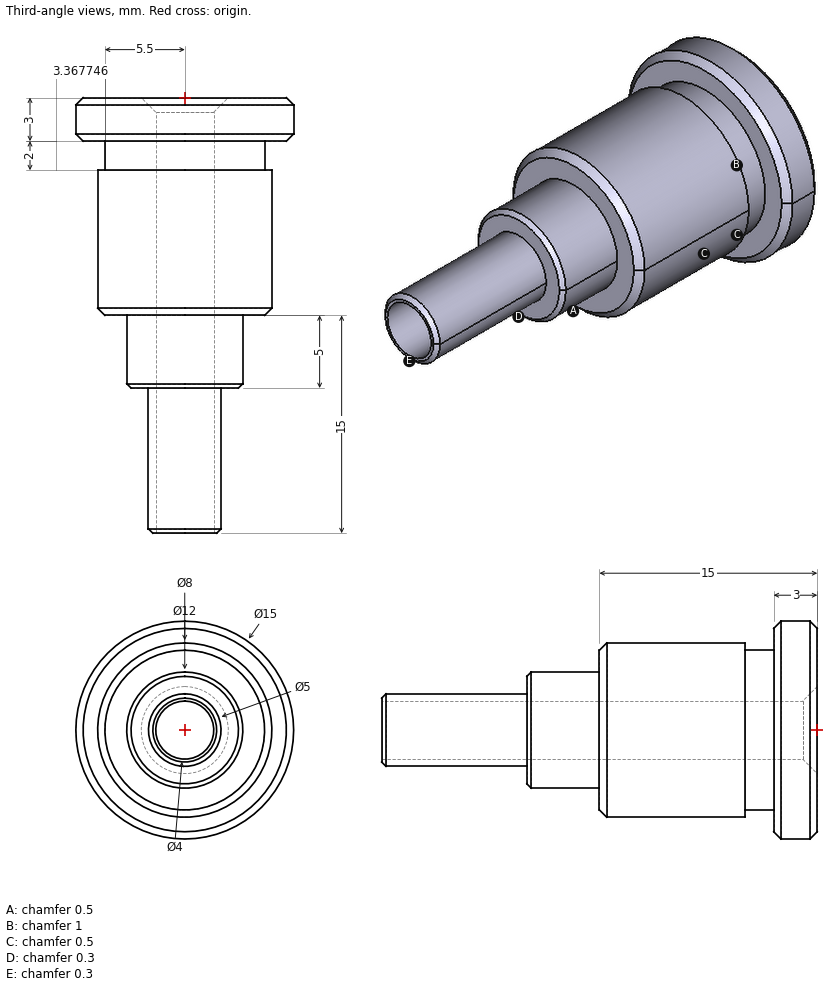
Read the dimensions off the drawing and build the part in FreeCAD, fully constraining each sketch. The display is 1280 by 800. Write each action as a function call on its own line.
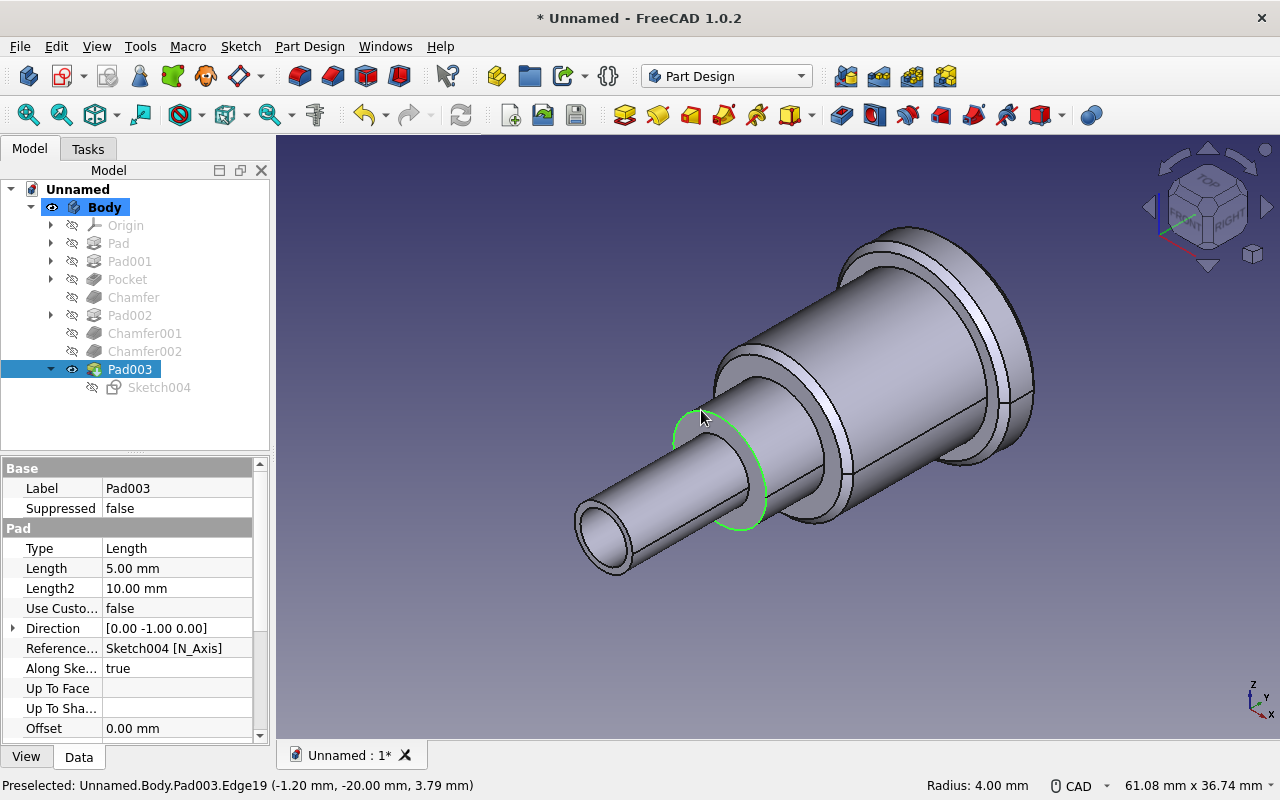
click(333, 76)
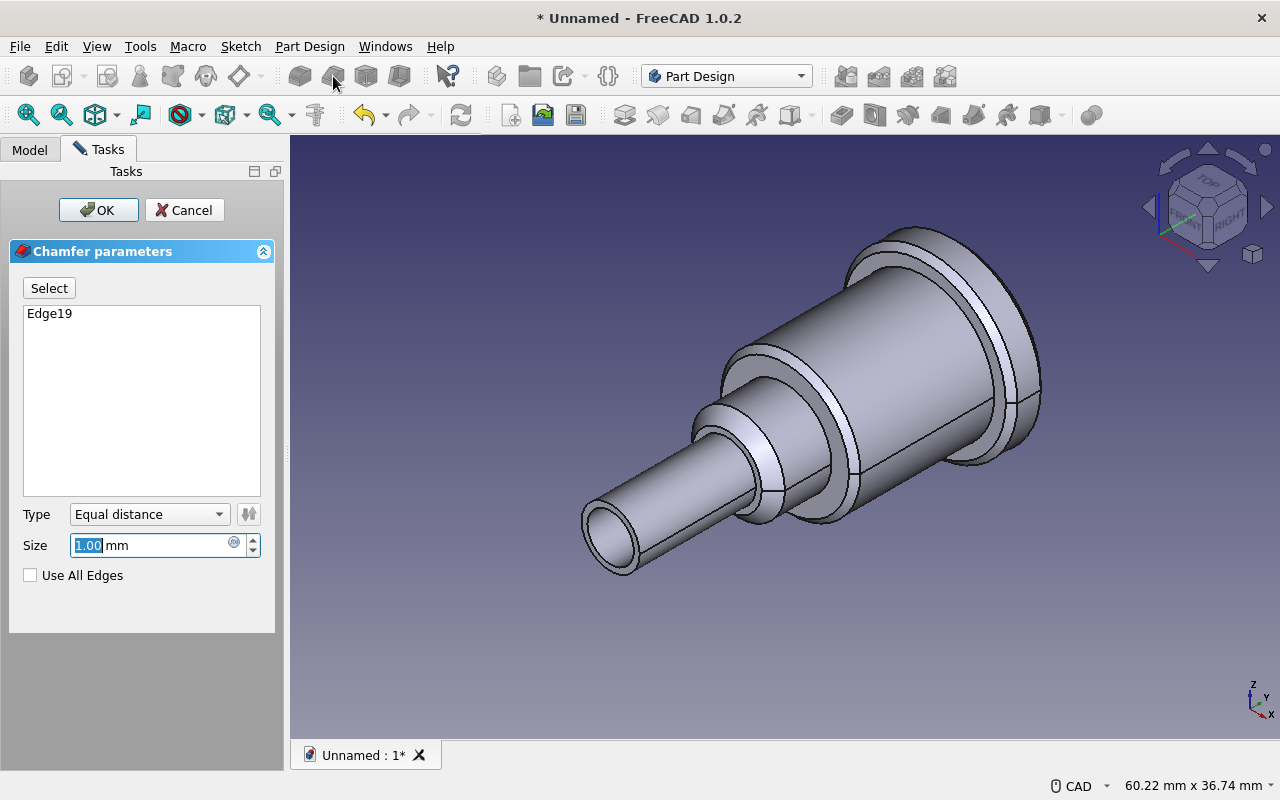
text(0.3)
key(Tab)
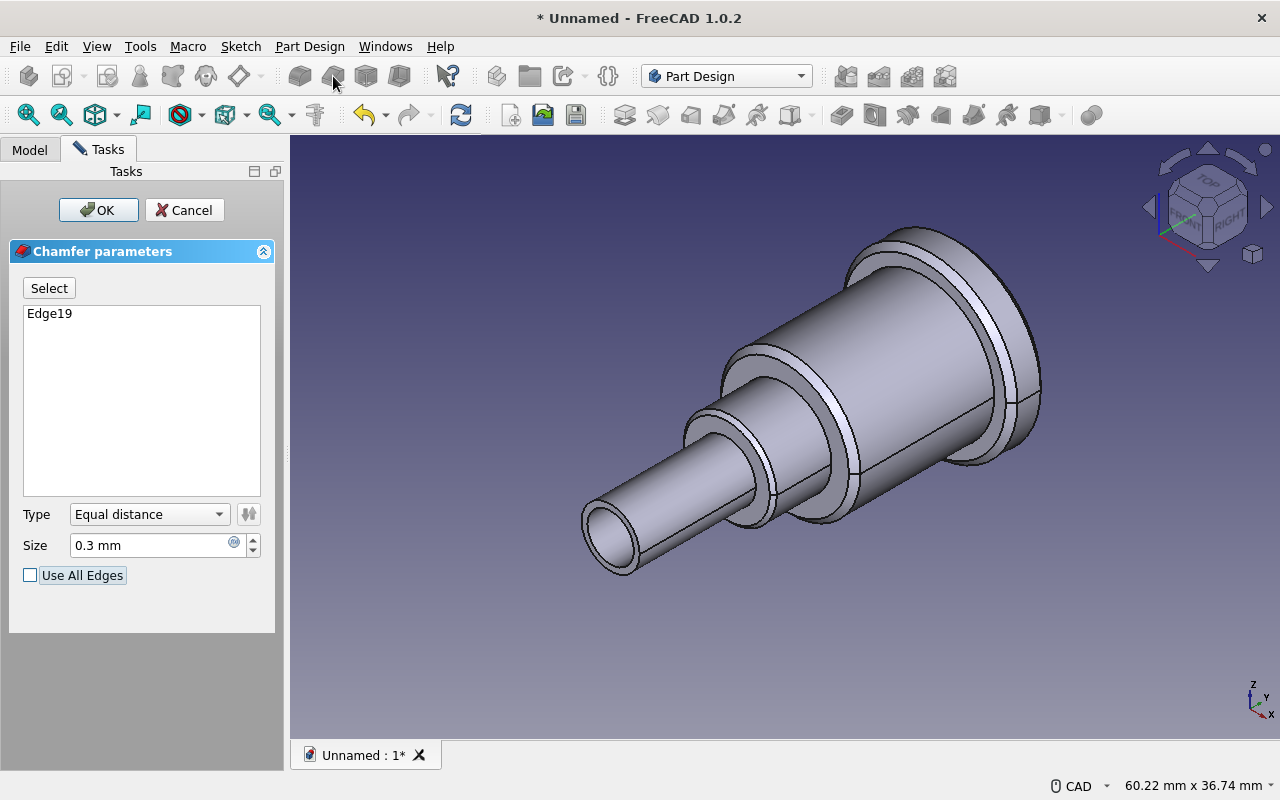
click(99, 210)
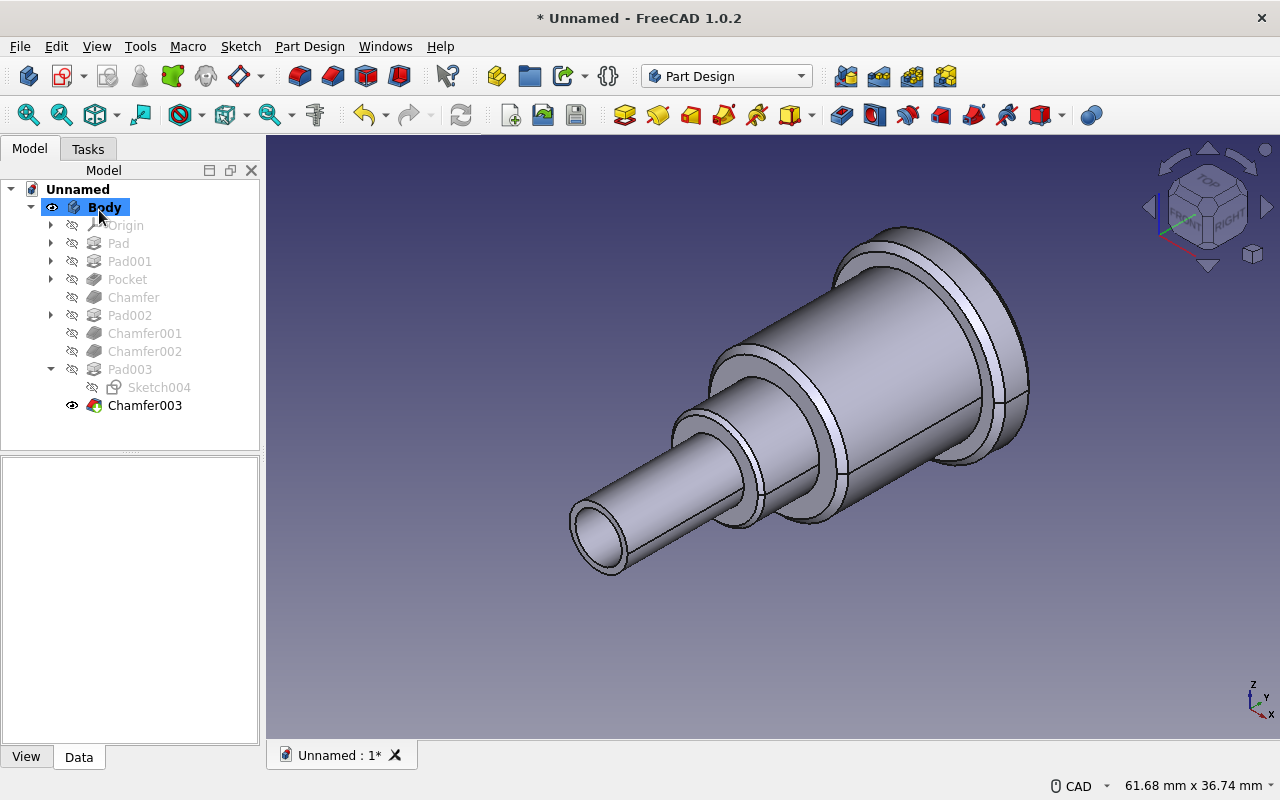
click(575, 503)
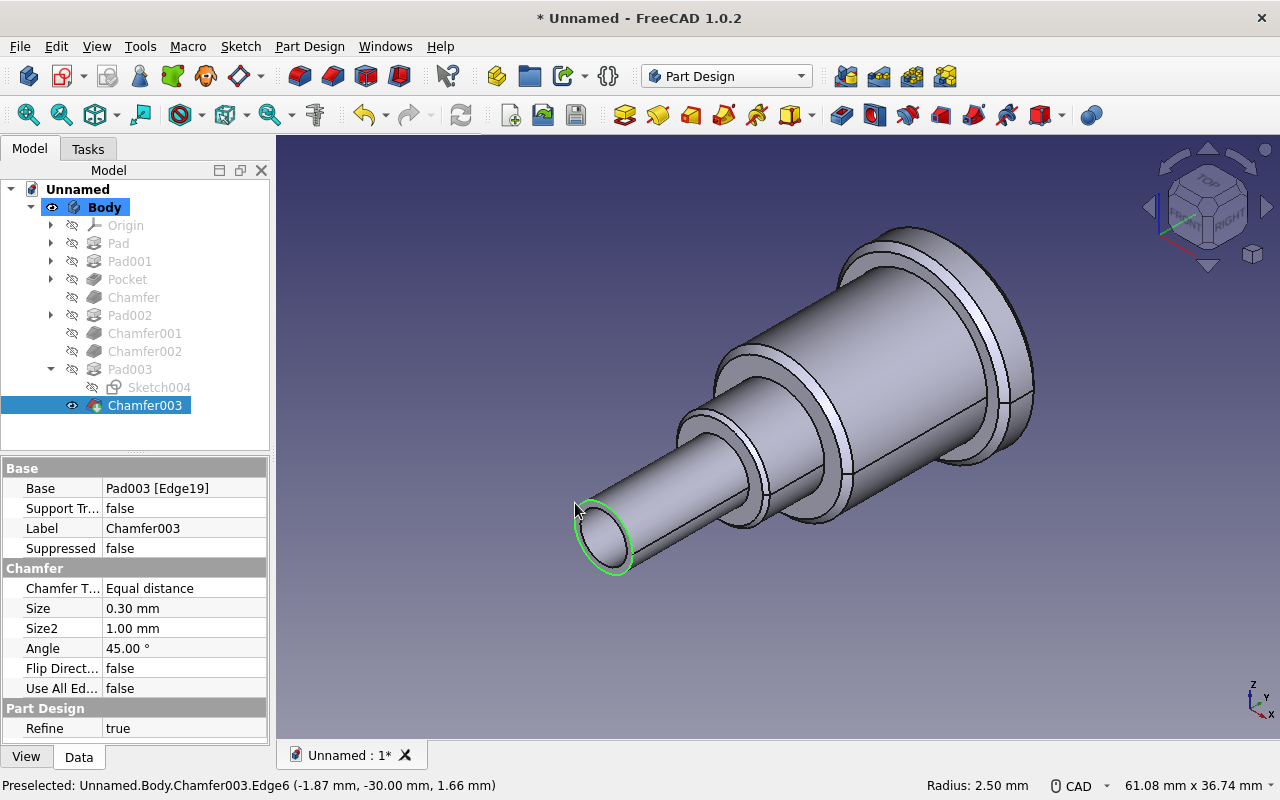
click(333, 76)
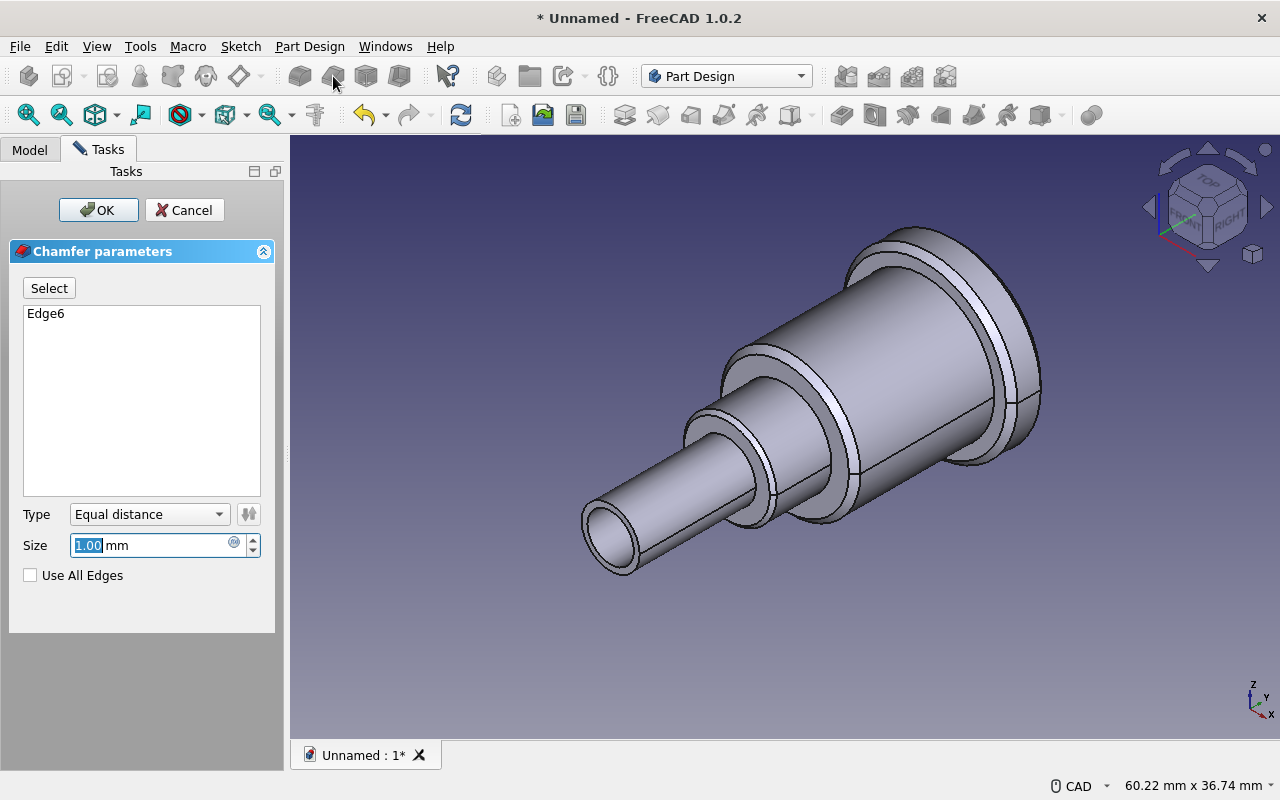
text(0.3)
key(Tab)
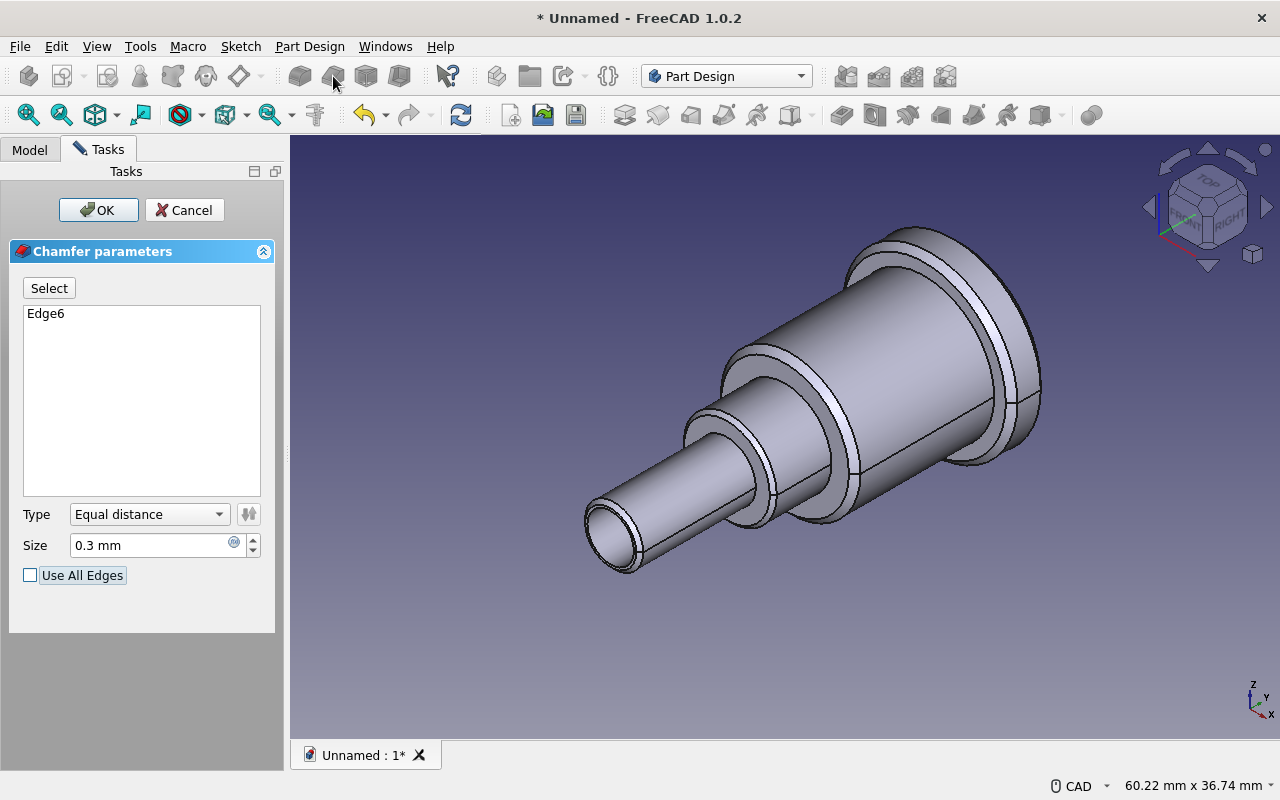
click(99, 210)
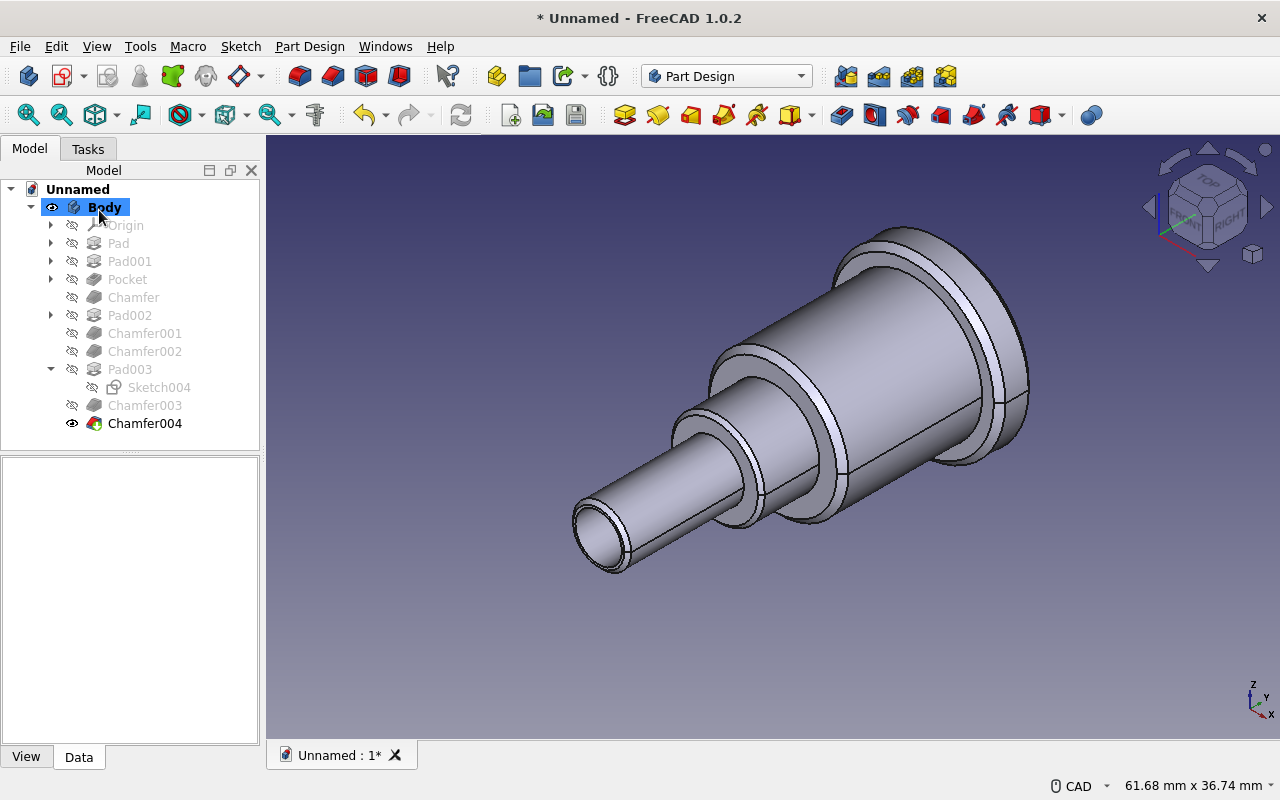
click(62, 76)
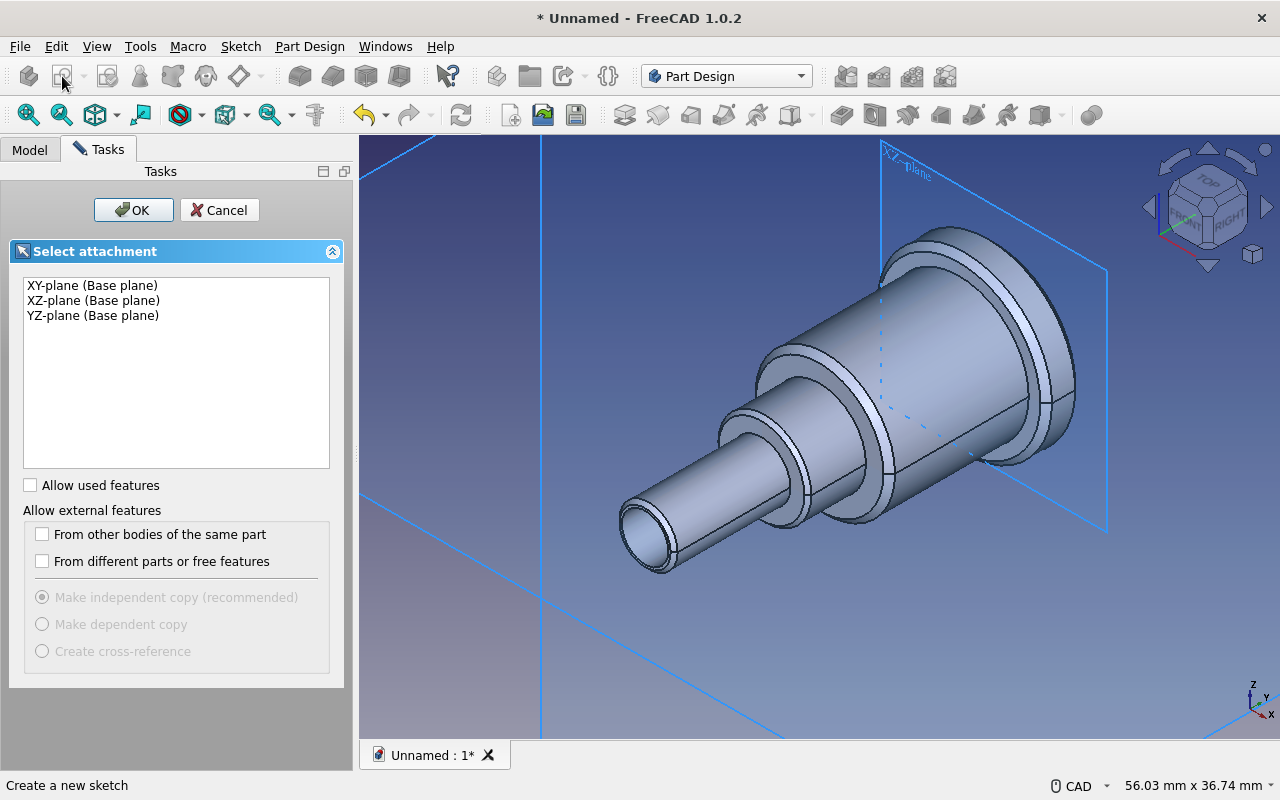
click(84, 286)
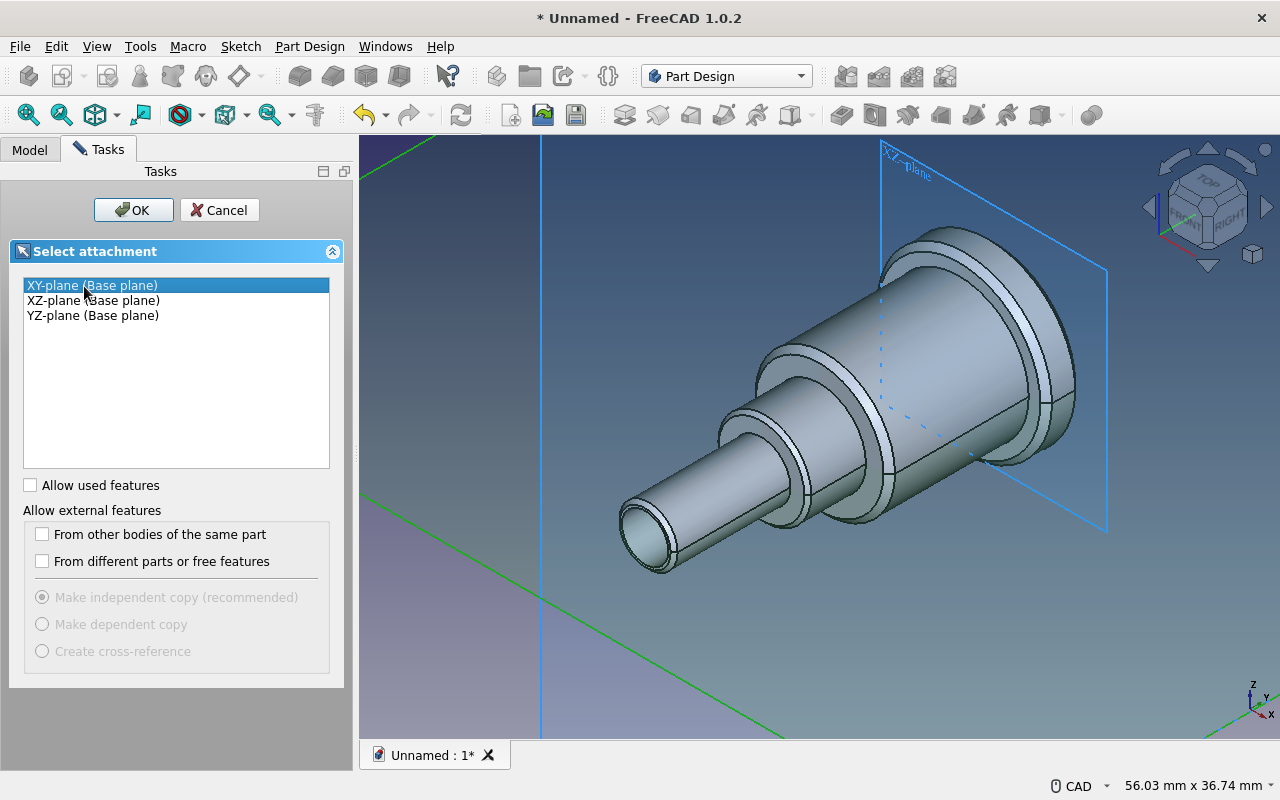
click(134, 210)